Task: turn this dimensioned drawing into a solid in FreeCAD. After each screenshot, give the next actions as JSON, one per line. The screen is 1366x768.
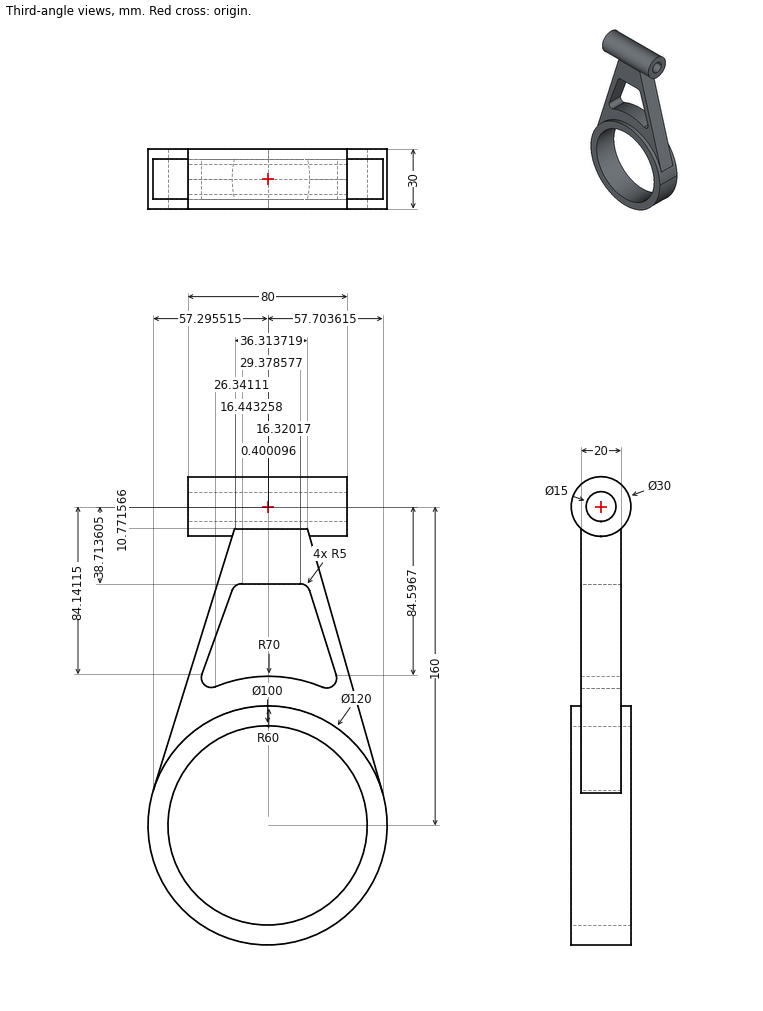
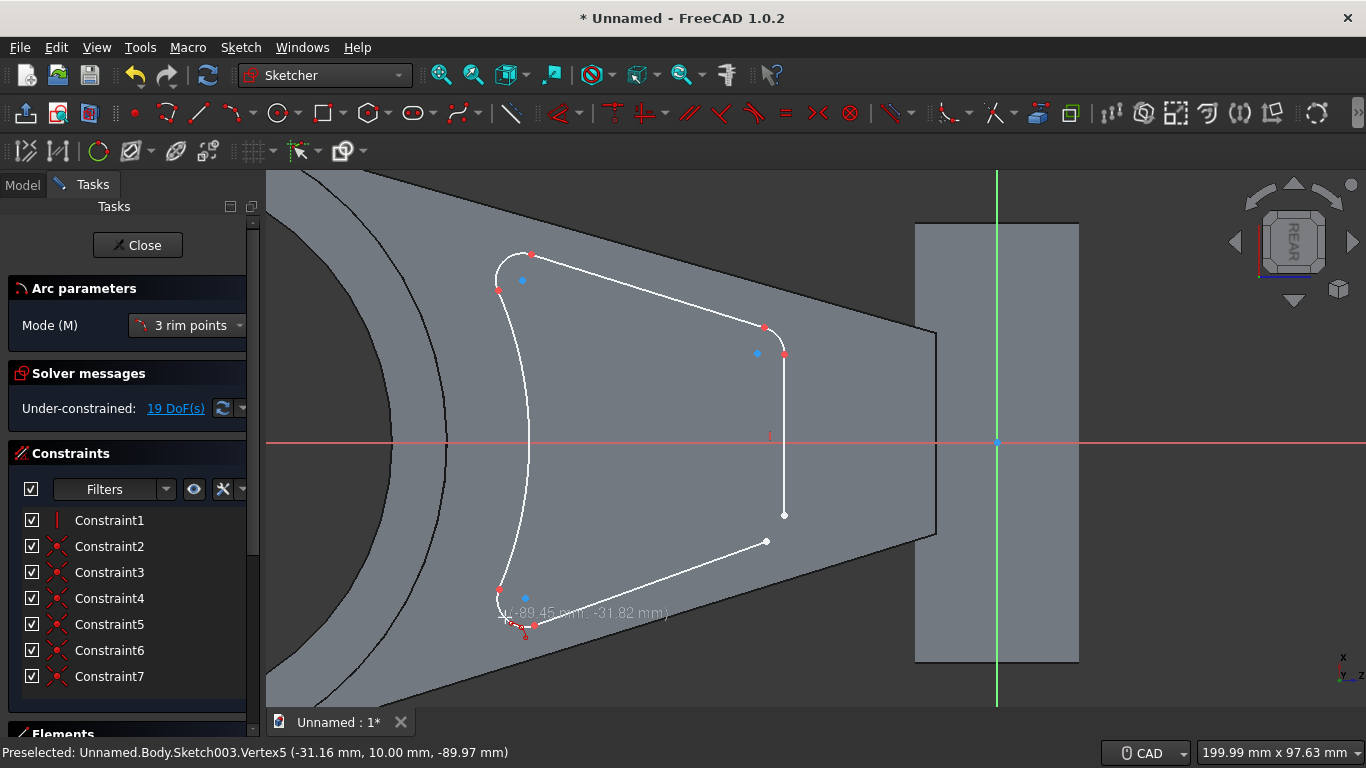
{"action": "left_click", "coordinate": [766, 542]}
{"action": "left_click", "coordinate": [784, 516]}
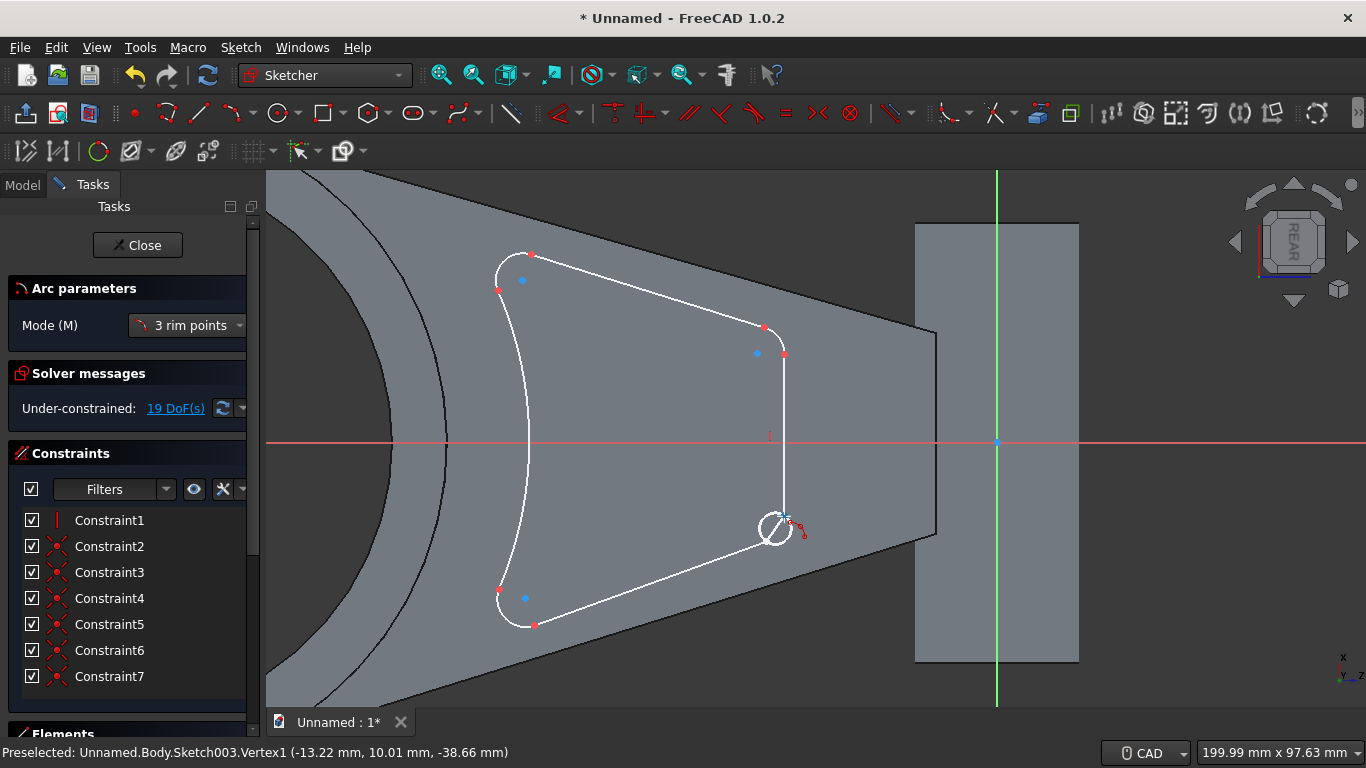
{"action": "scroll", "coordinate": [779, 531], "scroll_direction": "up", "scroll_amount": 6}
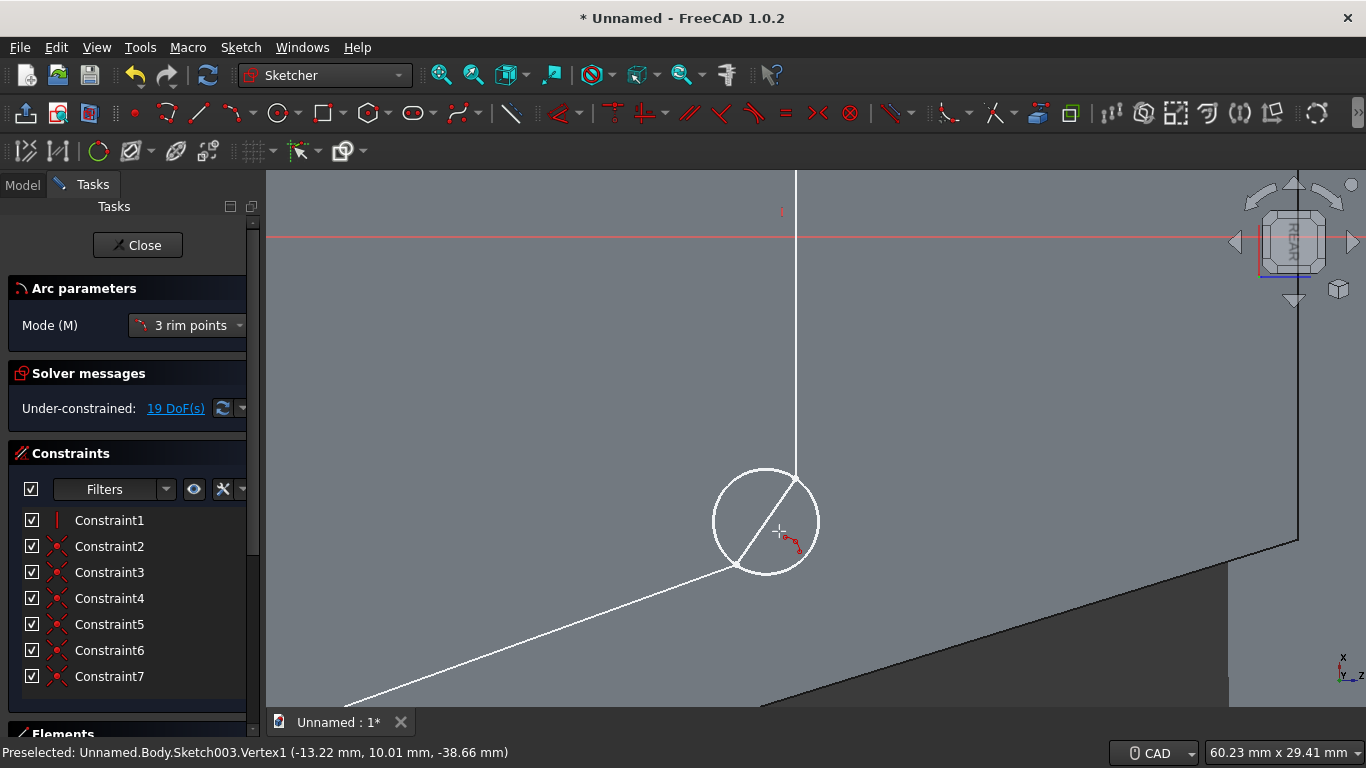
{"action": "left_click", "coordinate": [778, 528]}
{"action": "key", "text": "Escape"}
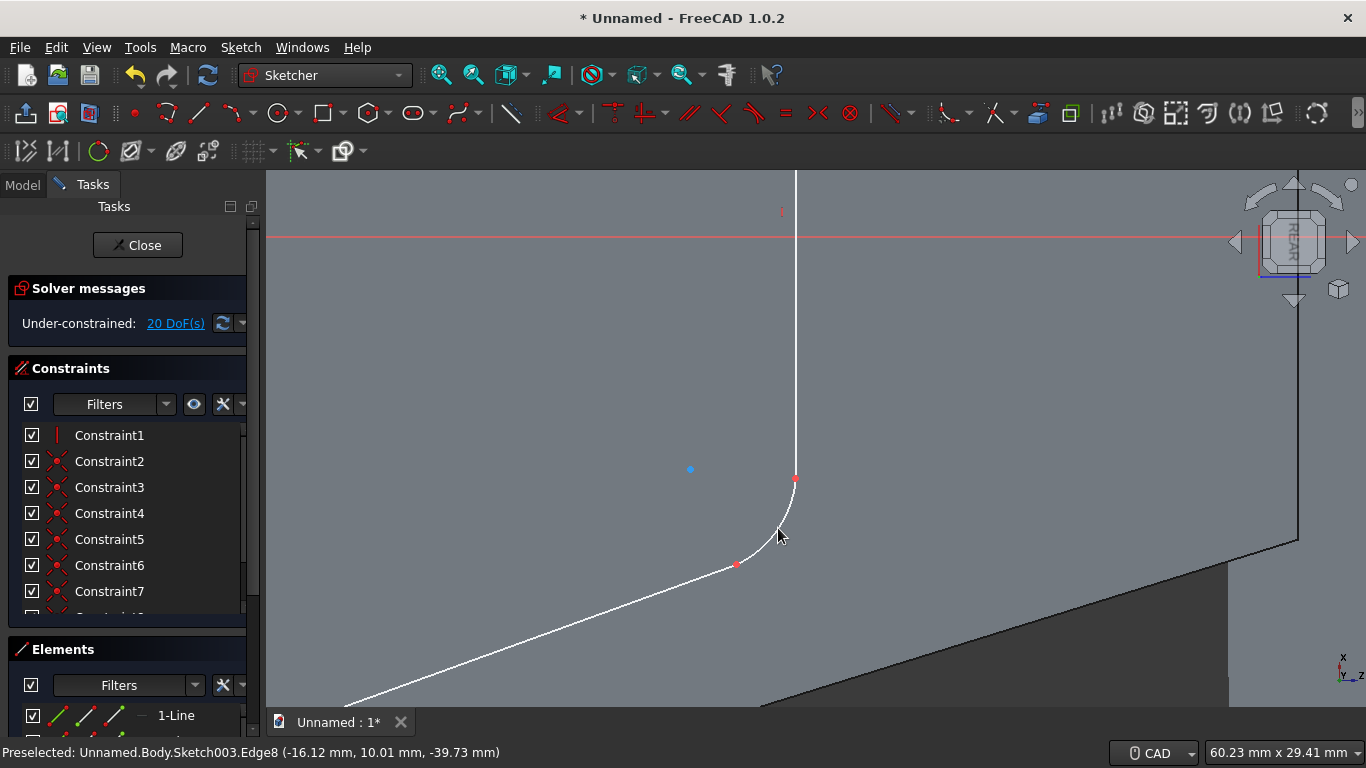
{"action": "left_click", "coordinate": [796, 318]}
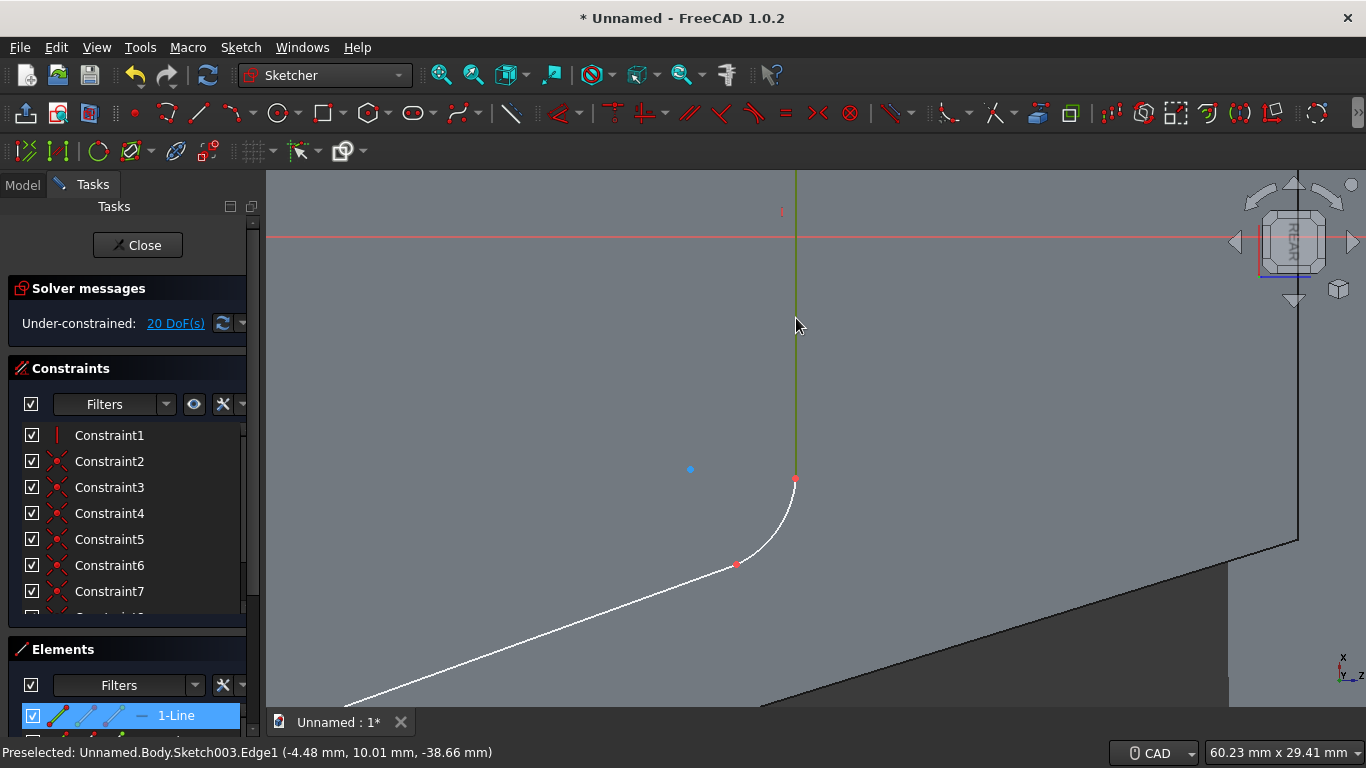
{"action": "scroll", "coordinate": [779, 531], "scroll_direction": "down", "scroll_amount": 6}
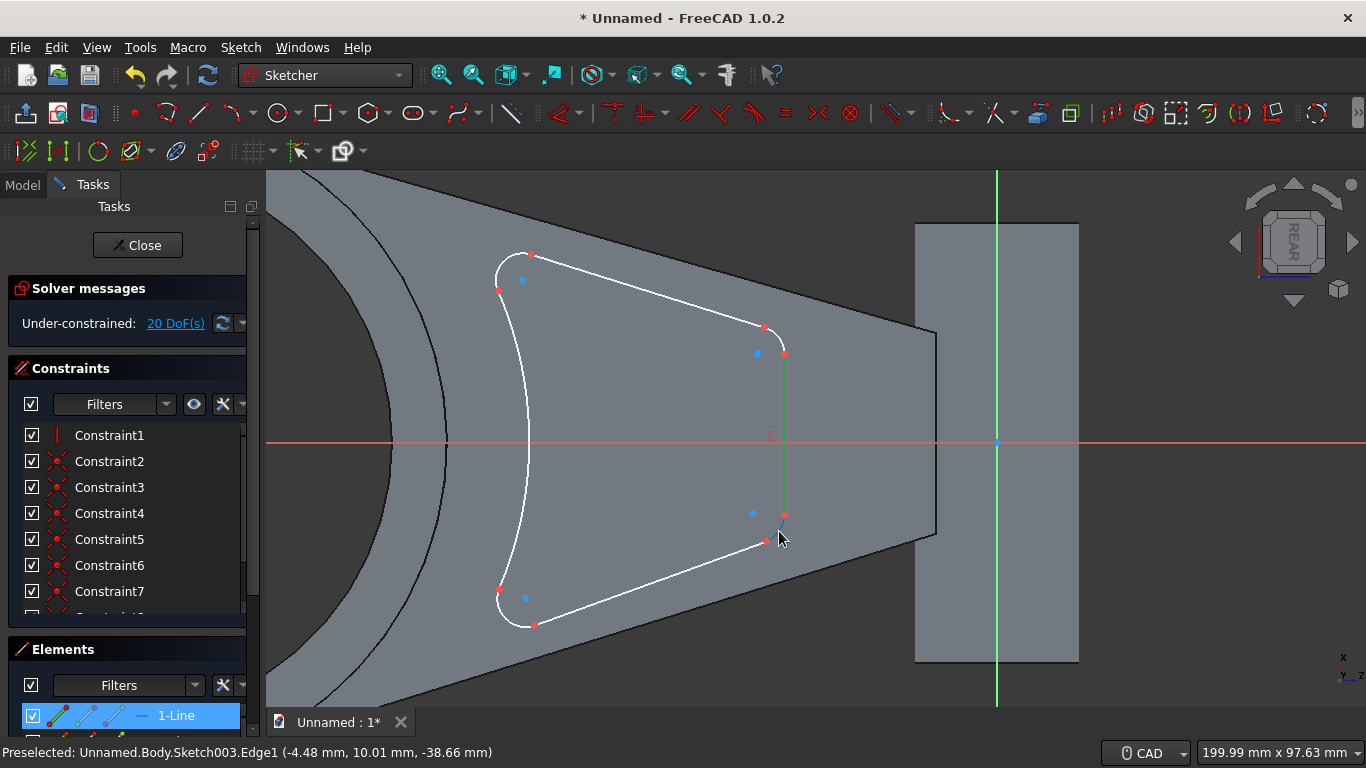
{"action": "scroll", "coordinate": [783, 344], "scroll_direction": "up", "scroll_amount": 2}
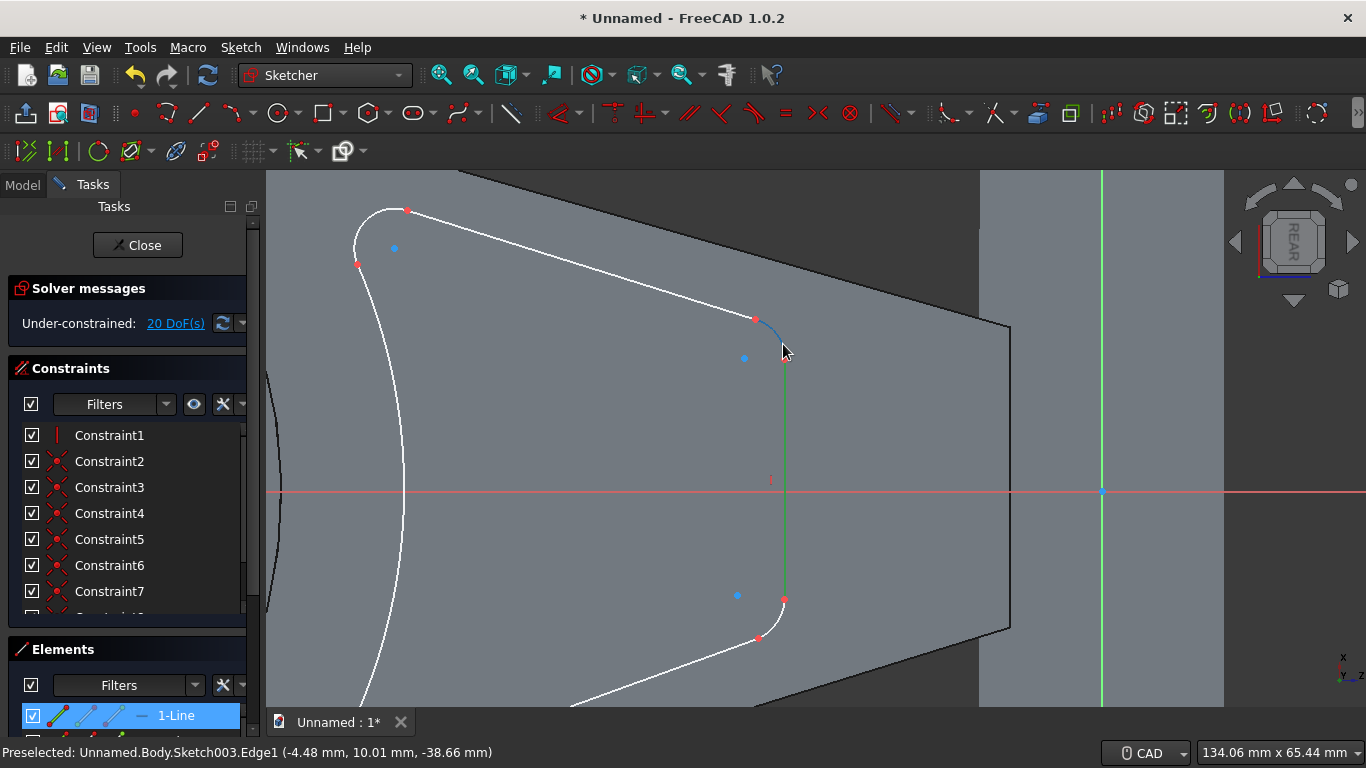
{"action": "left_click", "coordinate": [782, 344]}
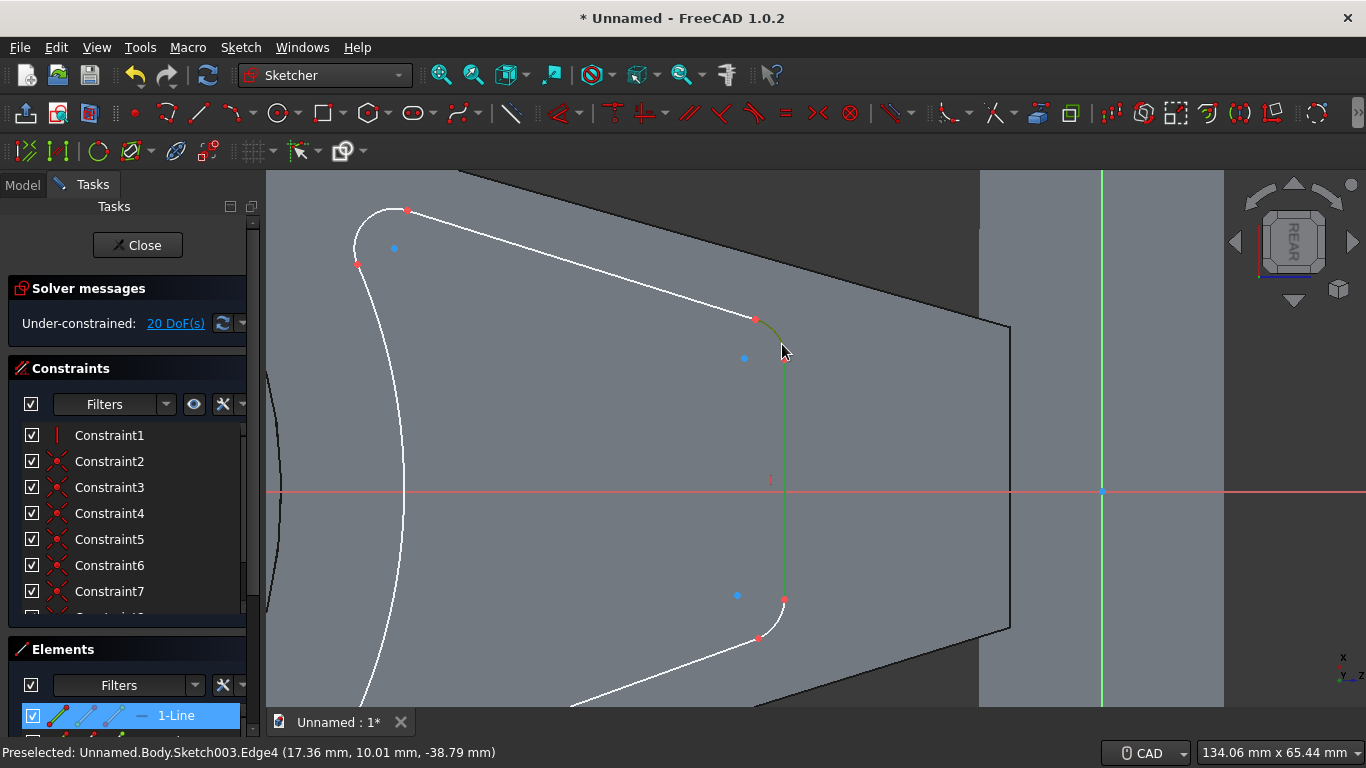
{"action": "left_click", "coordinate": [754, 114]}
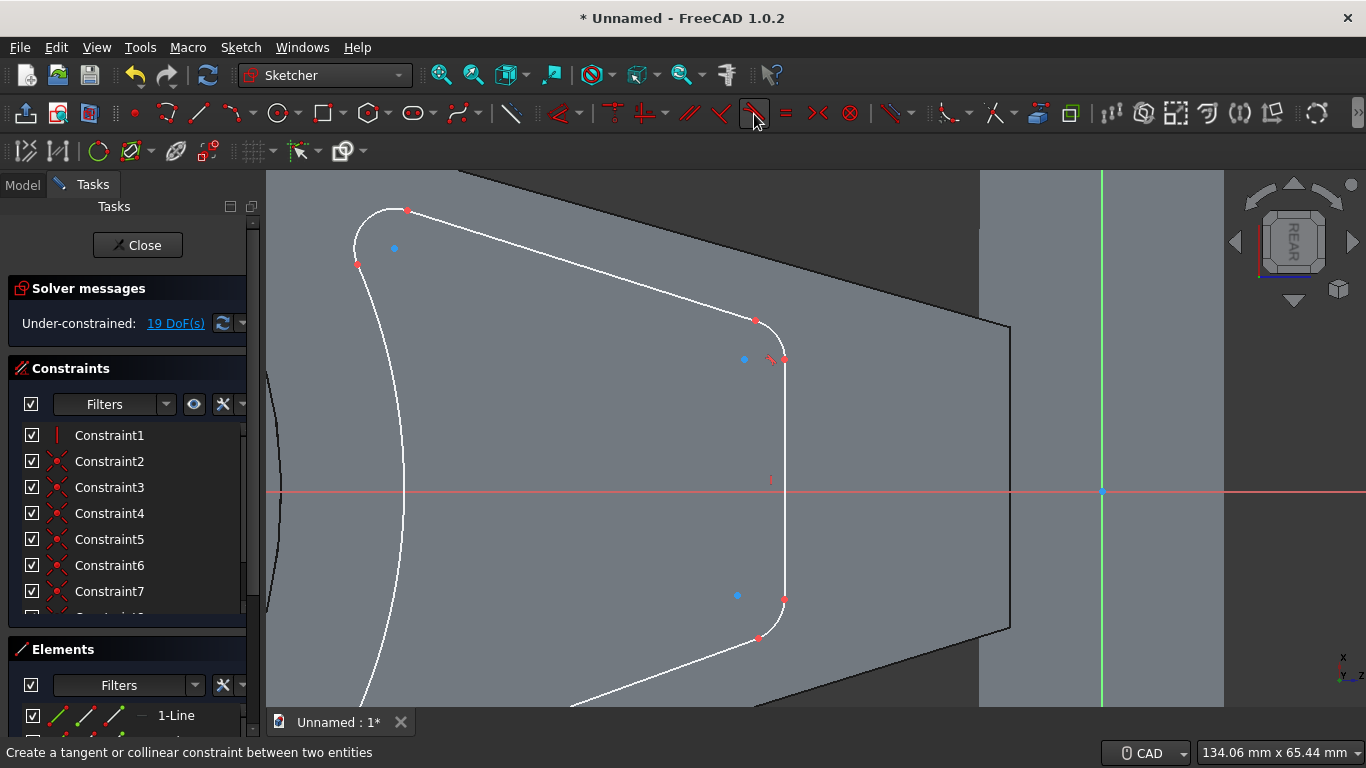
{"action": "left_click", "coordinate": [785, 528]}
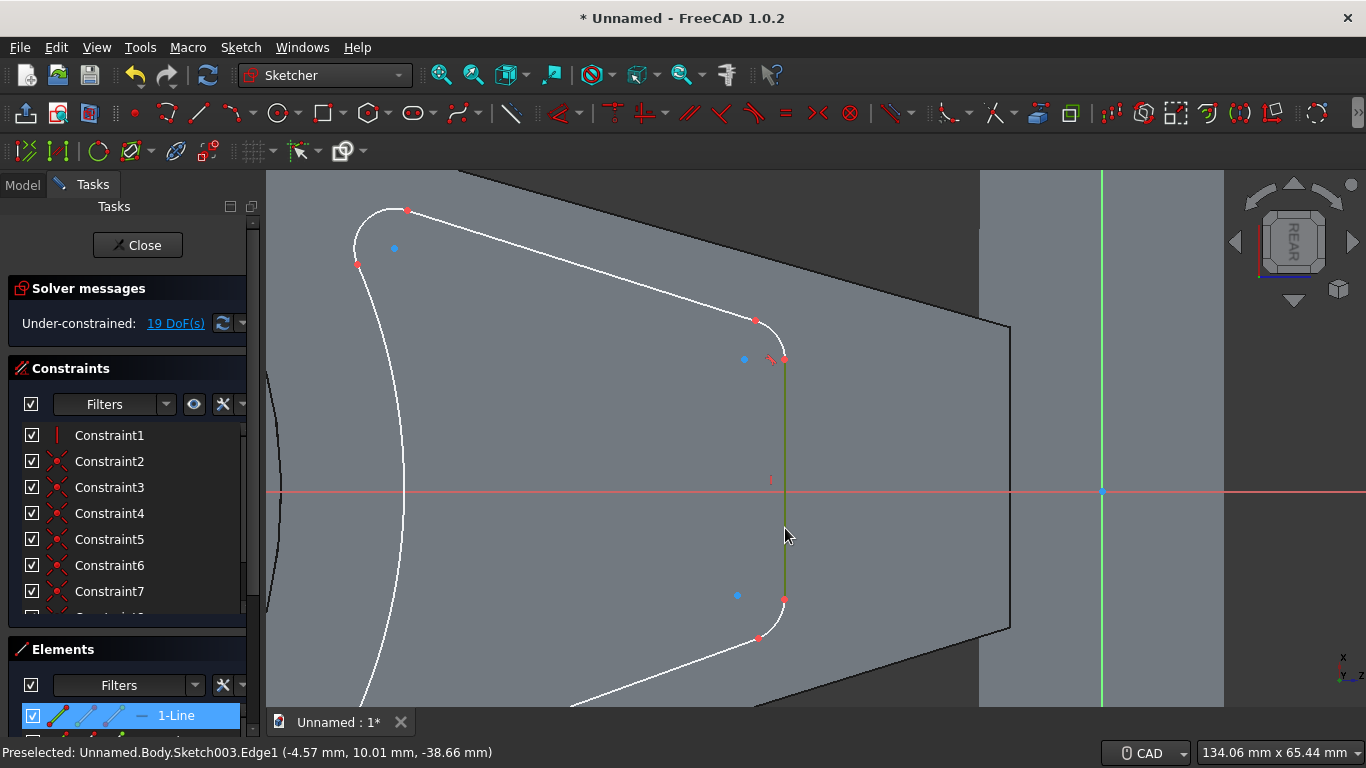
{"action": "left_click", "coordinate": [770, 630]}